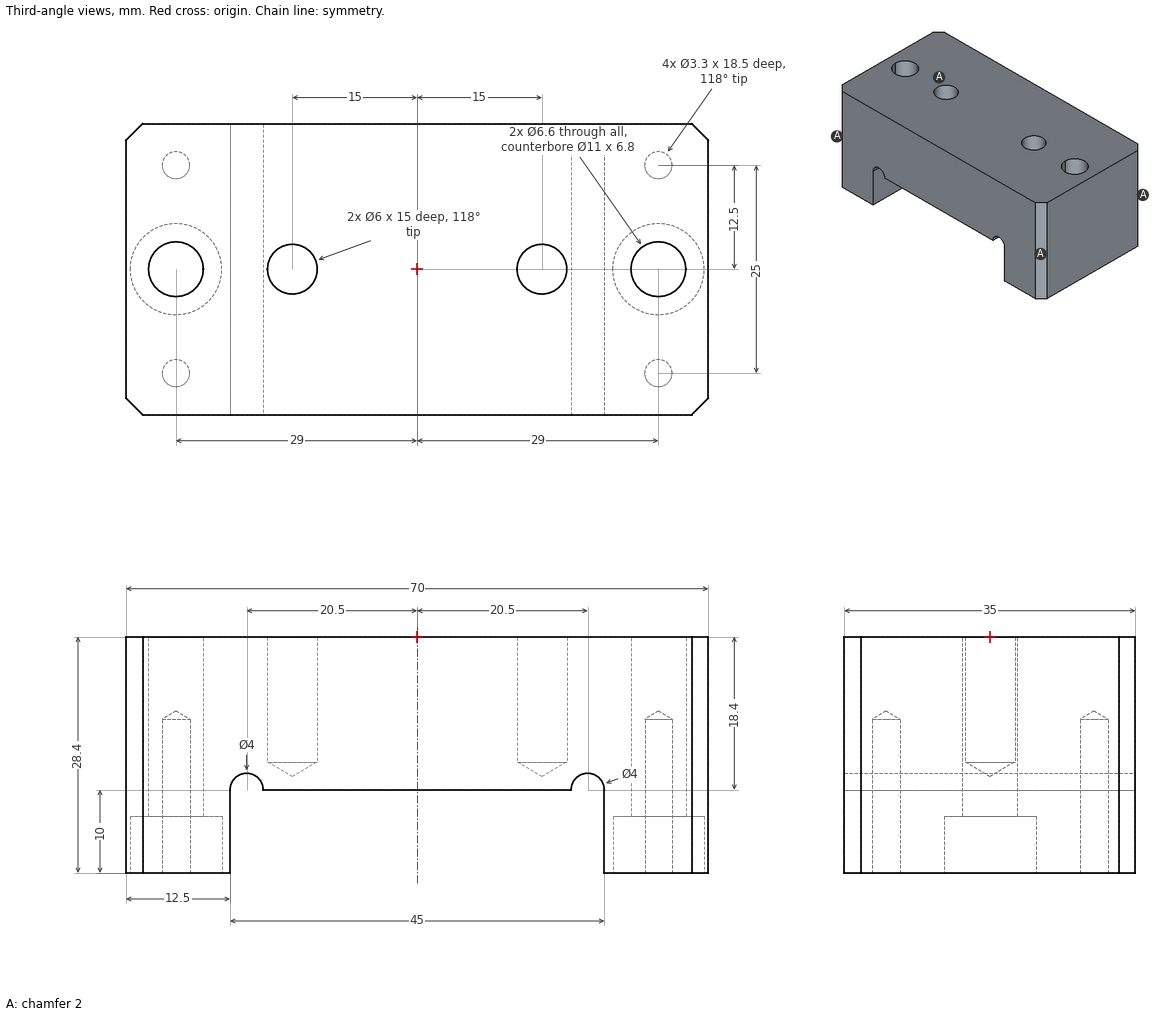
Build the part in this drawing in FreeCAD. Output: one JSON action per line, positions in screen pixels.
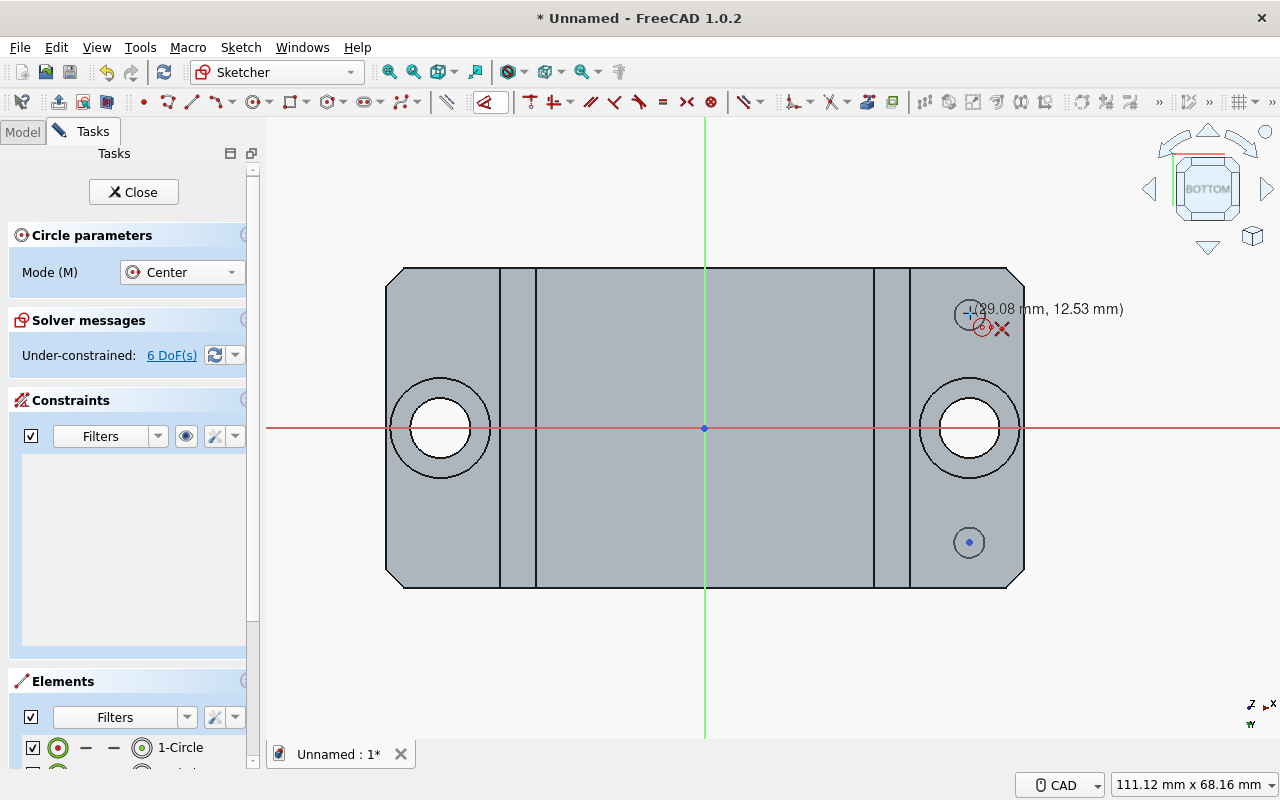
{"action": "scroll", "coordinate": [440, 542], "scroll_direction": "up", "scroll_amount": 3}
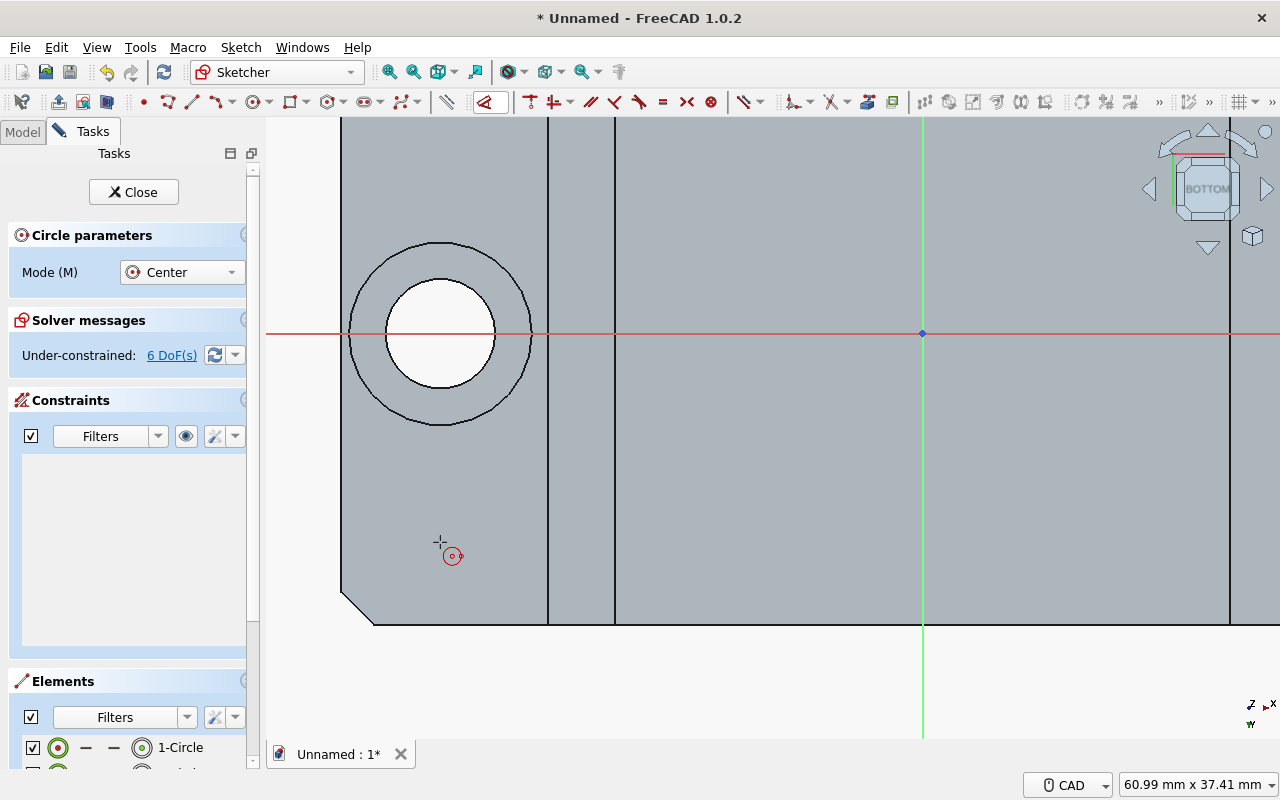
{"action": "left_click", "coordinate": [440, 542]}
{"action": "left_click", "coordinate": [460, 522]}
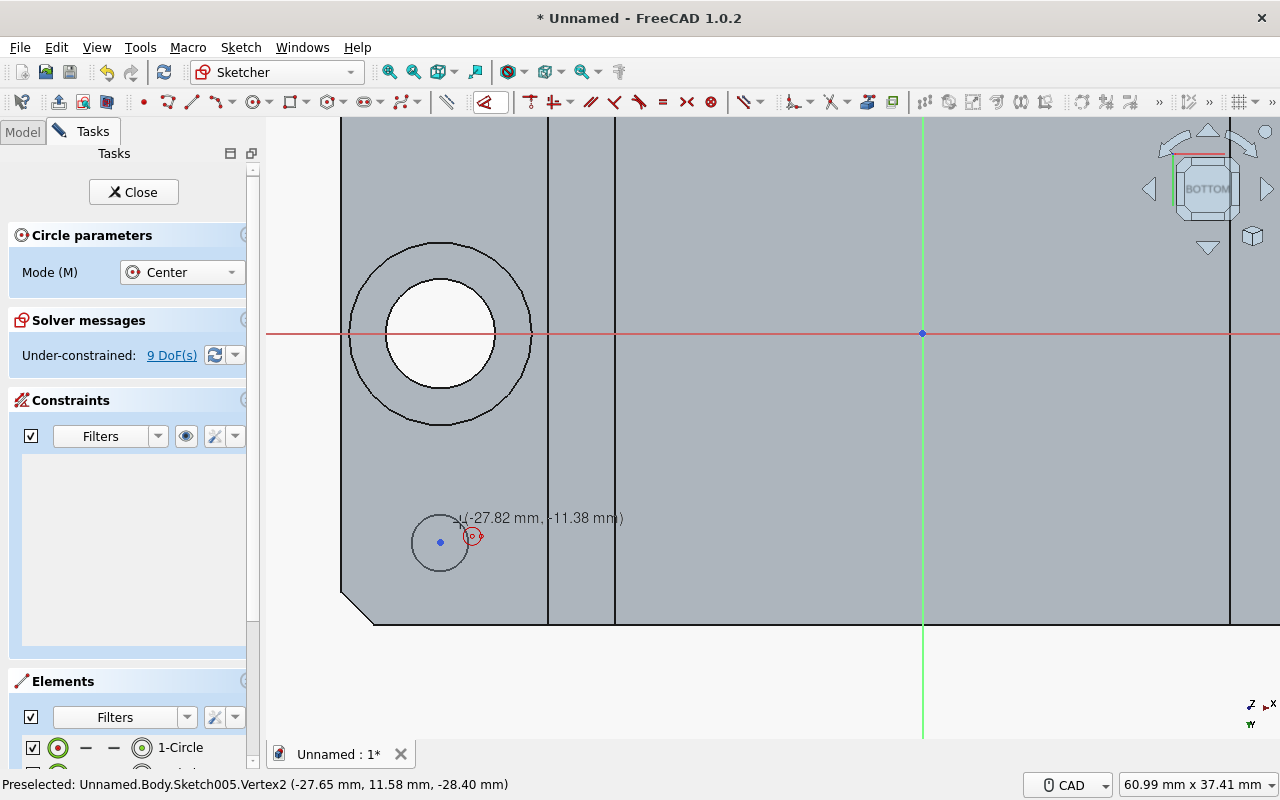
{"action": "scroll", "coordinate": [439, 543], "scroll_direction": "down", "scroll_amount": 3}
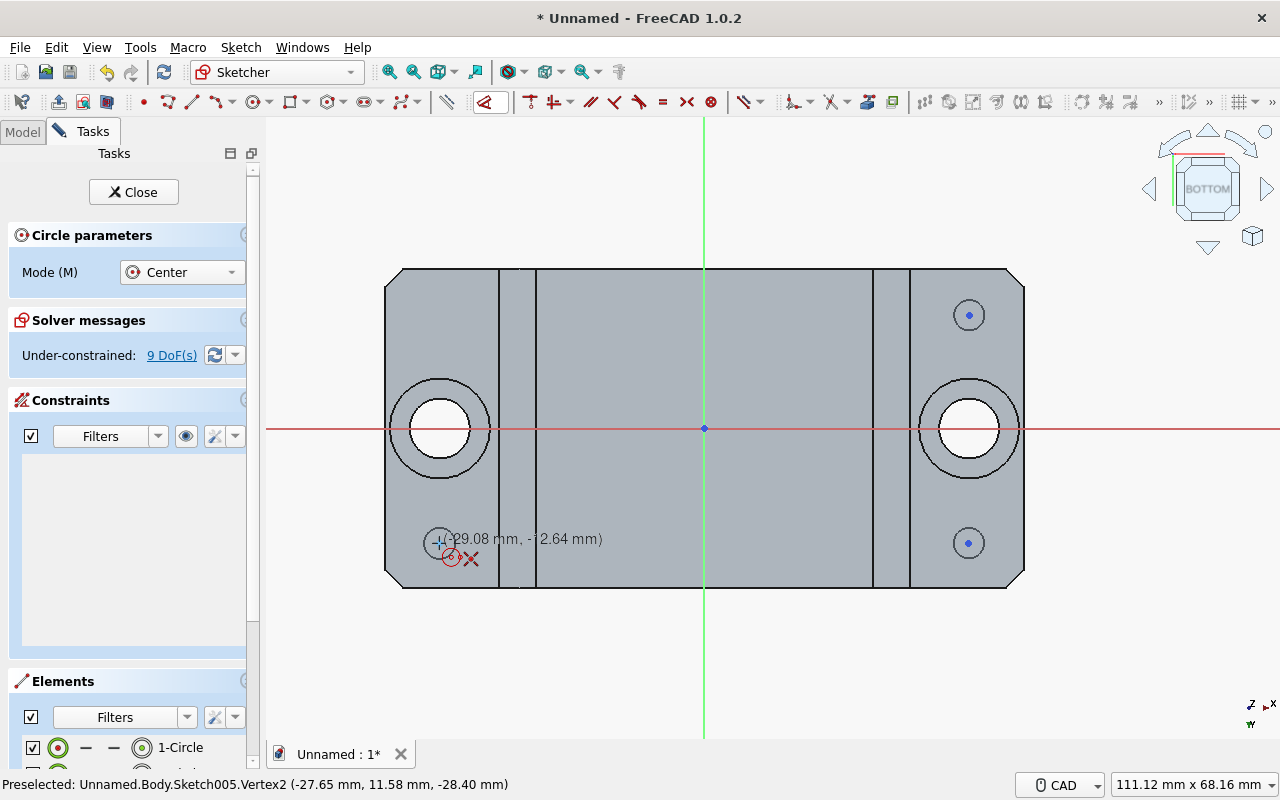
{"action": "scroll", "coordinate": [440, 314], "scroll_direction": "up", "scroll_amount": 3}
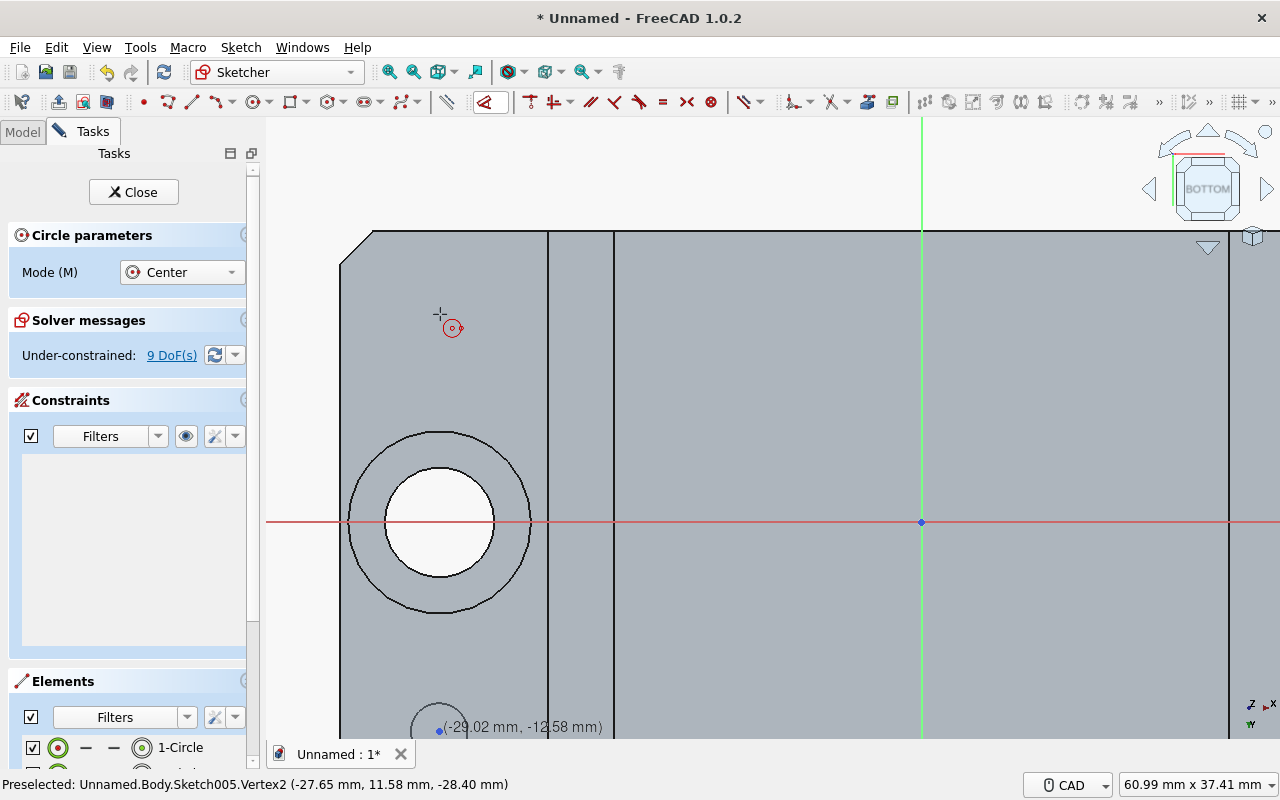
{"action": "left_click", "coordinate": [440, 315]}
{"action": "left_click", "coordinate": [459, 295]}
{"action": "key", "text": "Escape"}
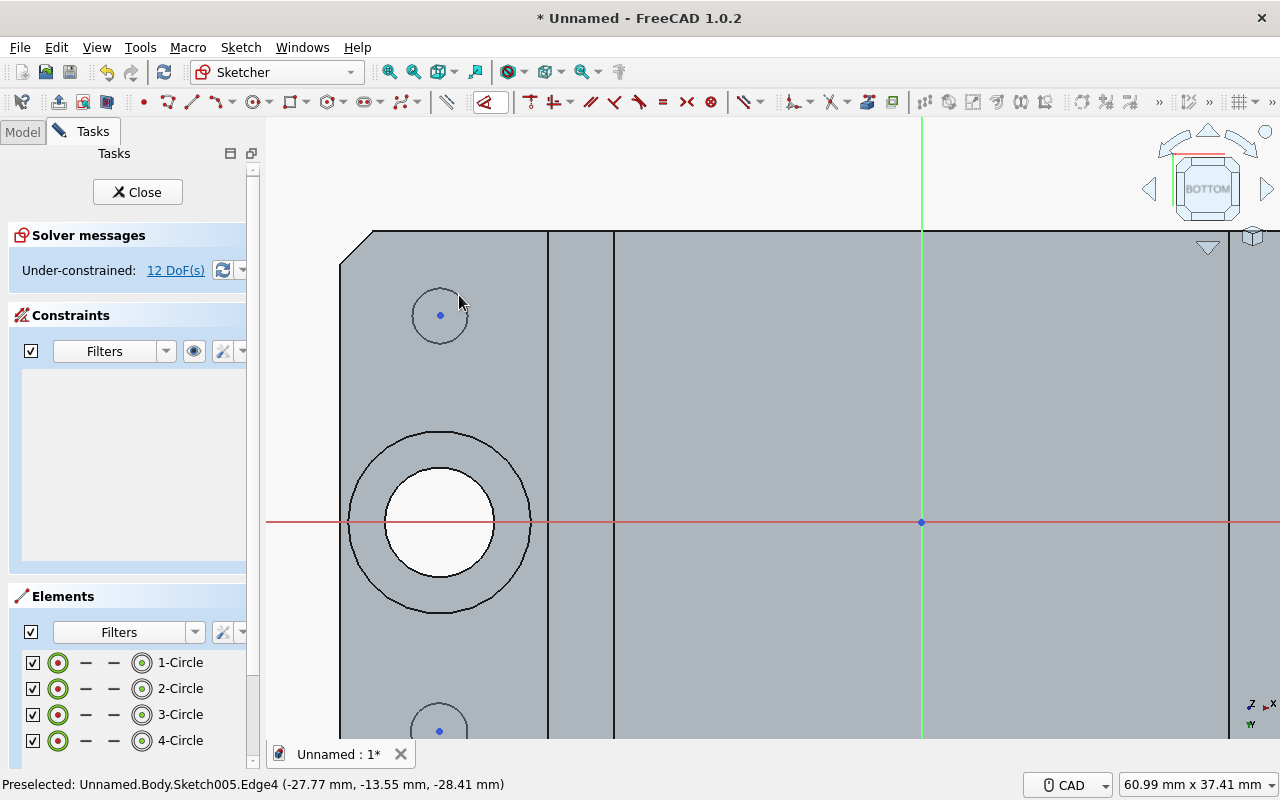
{"action": "scroll", "coordinate": [440, 313], "scroll_direction": "down", "scroll_amount": 3}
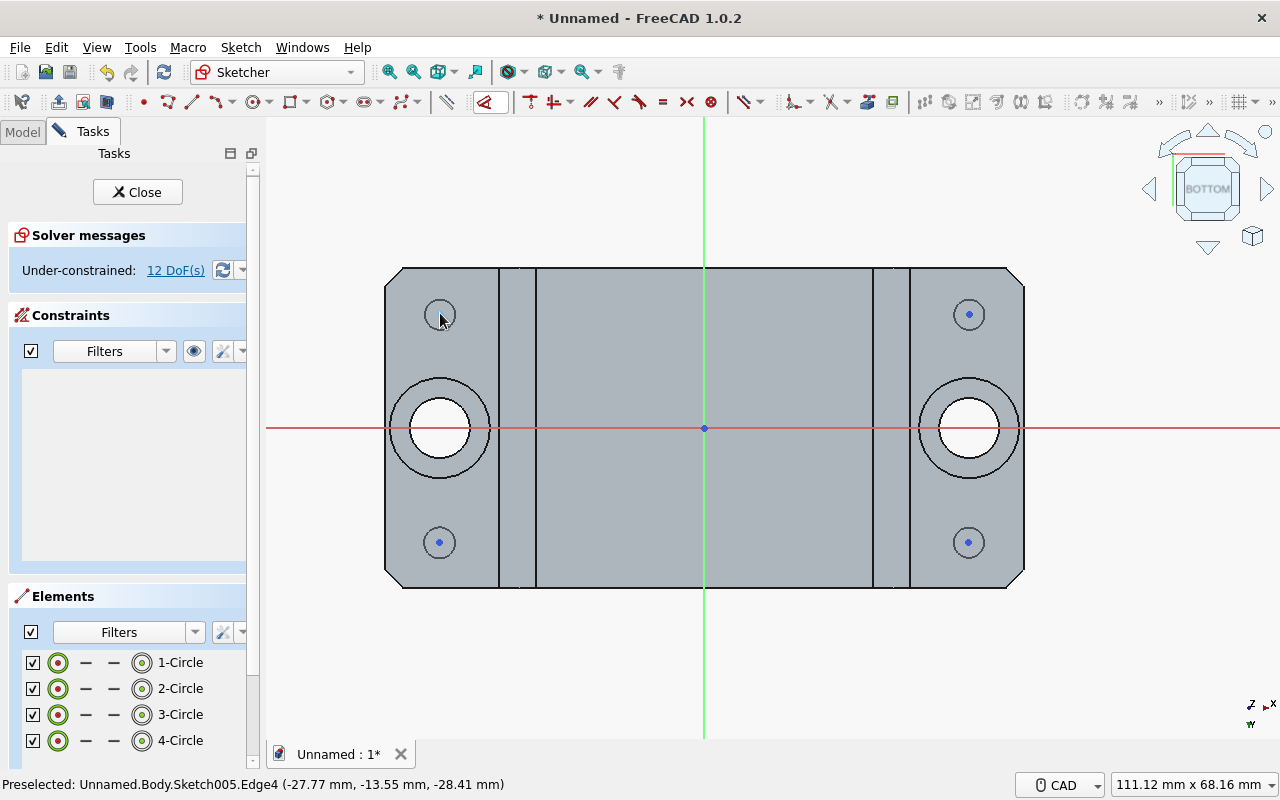
{"action": "left_click", "coordinate": [980, 532]}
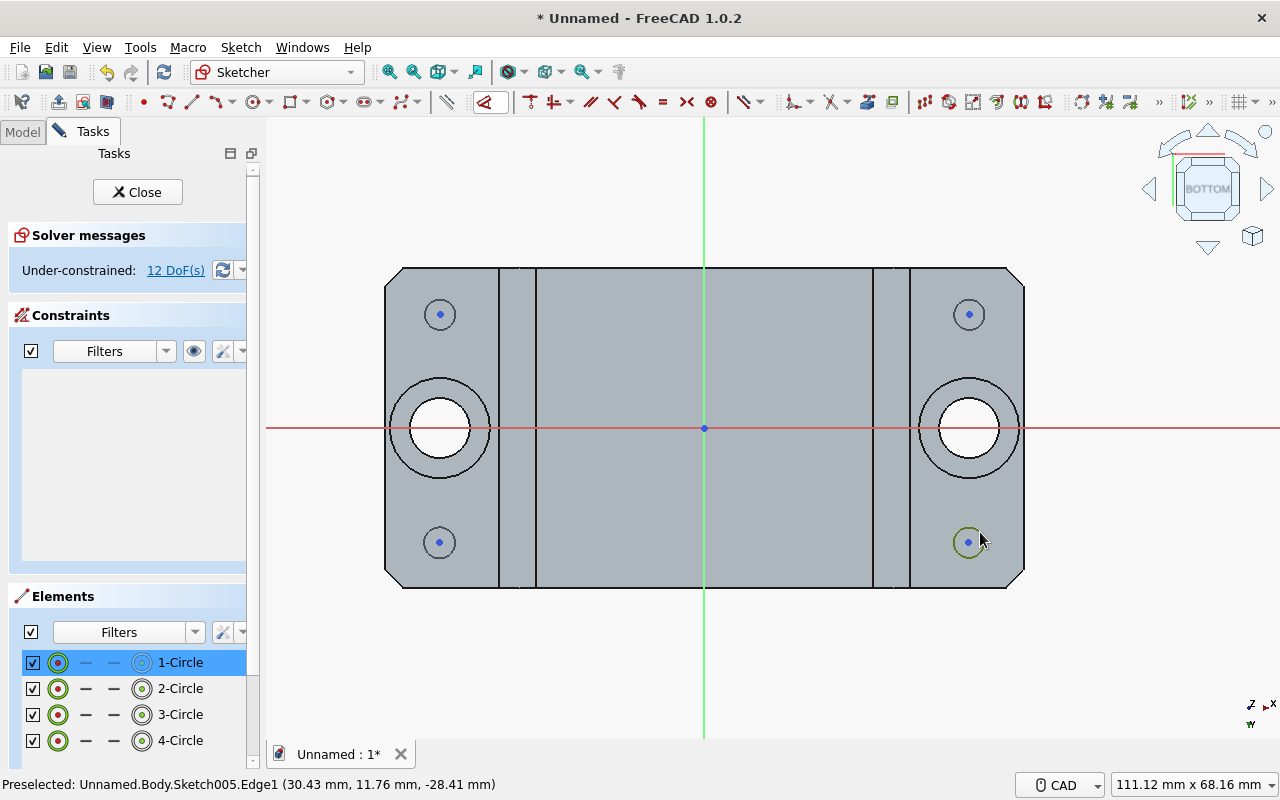
{"action": "left_click", "coordinate": [980, 304]}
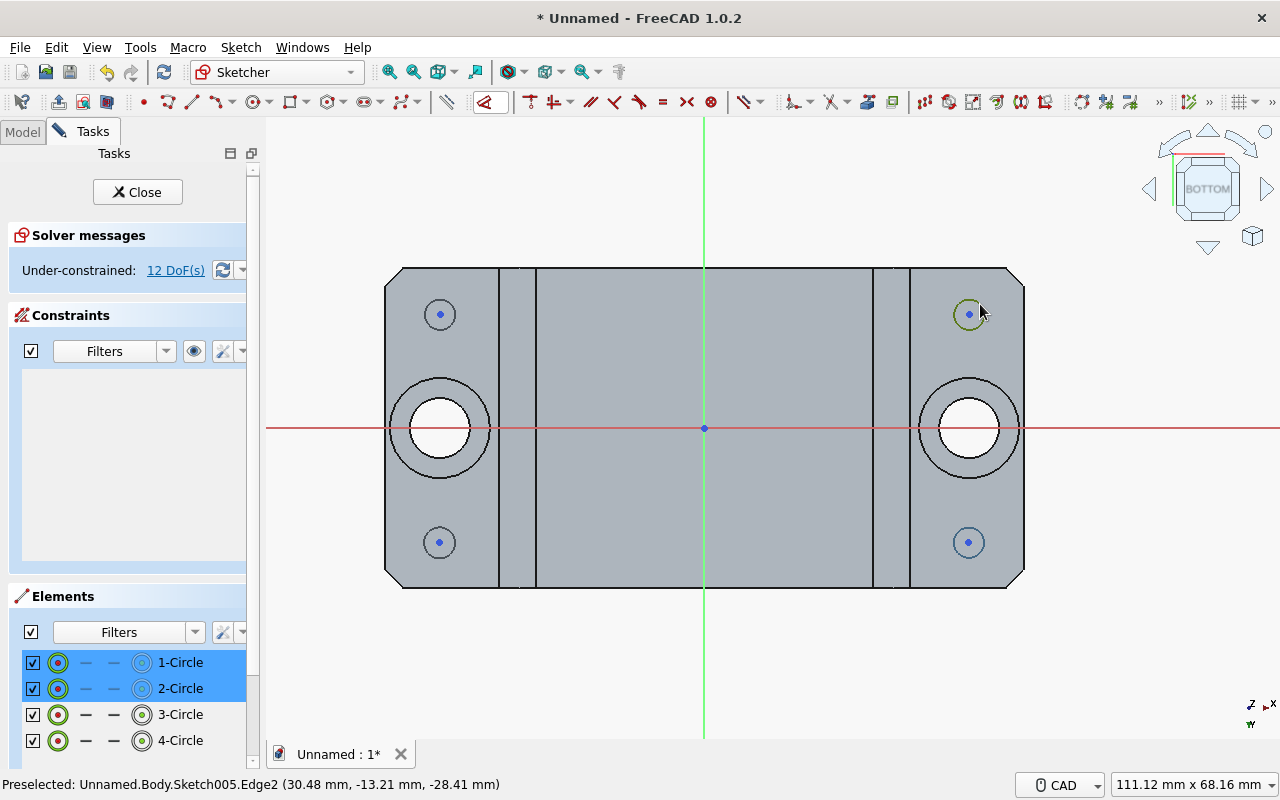
{"action": "left_click", "coordinate": [451, 532]}